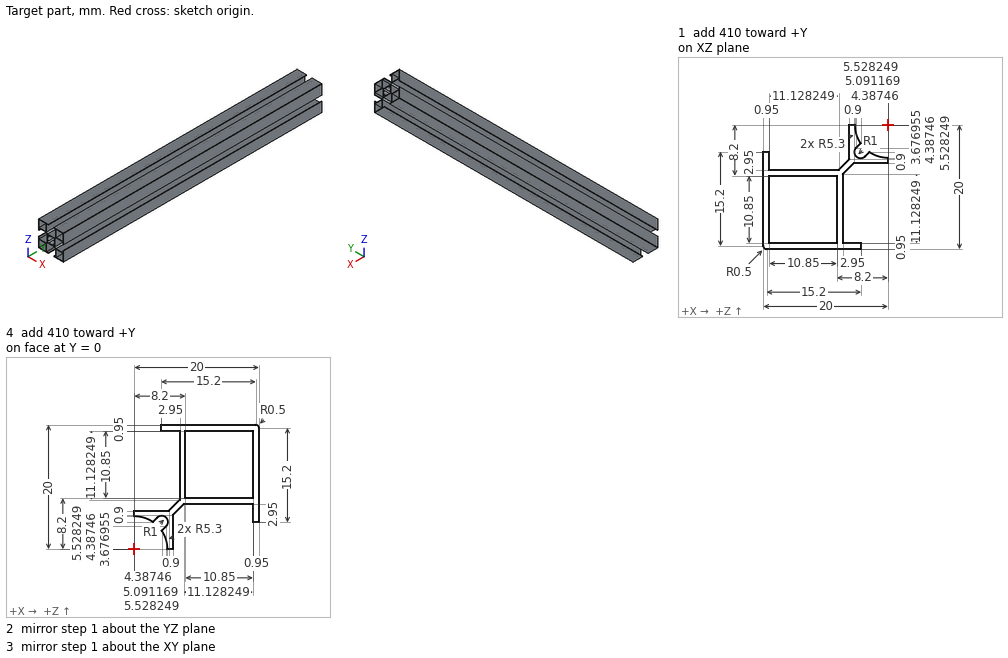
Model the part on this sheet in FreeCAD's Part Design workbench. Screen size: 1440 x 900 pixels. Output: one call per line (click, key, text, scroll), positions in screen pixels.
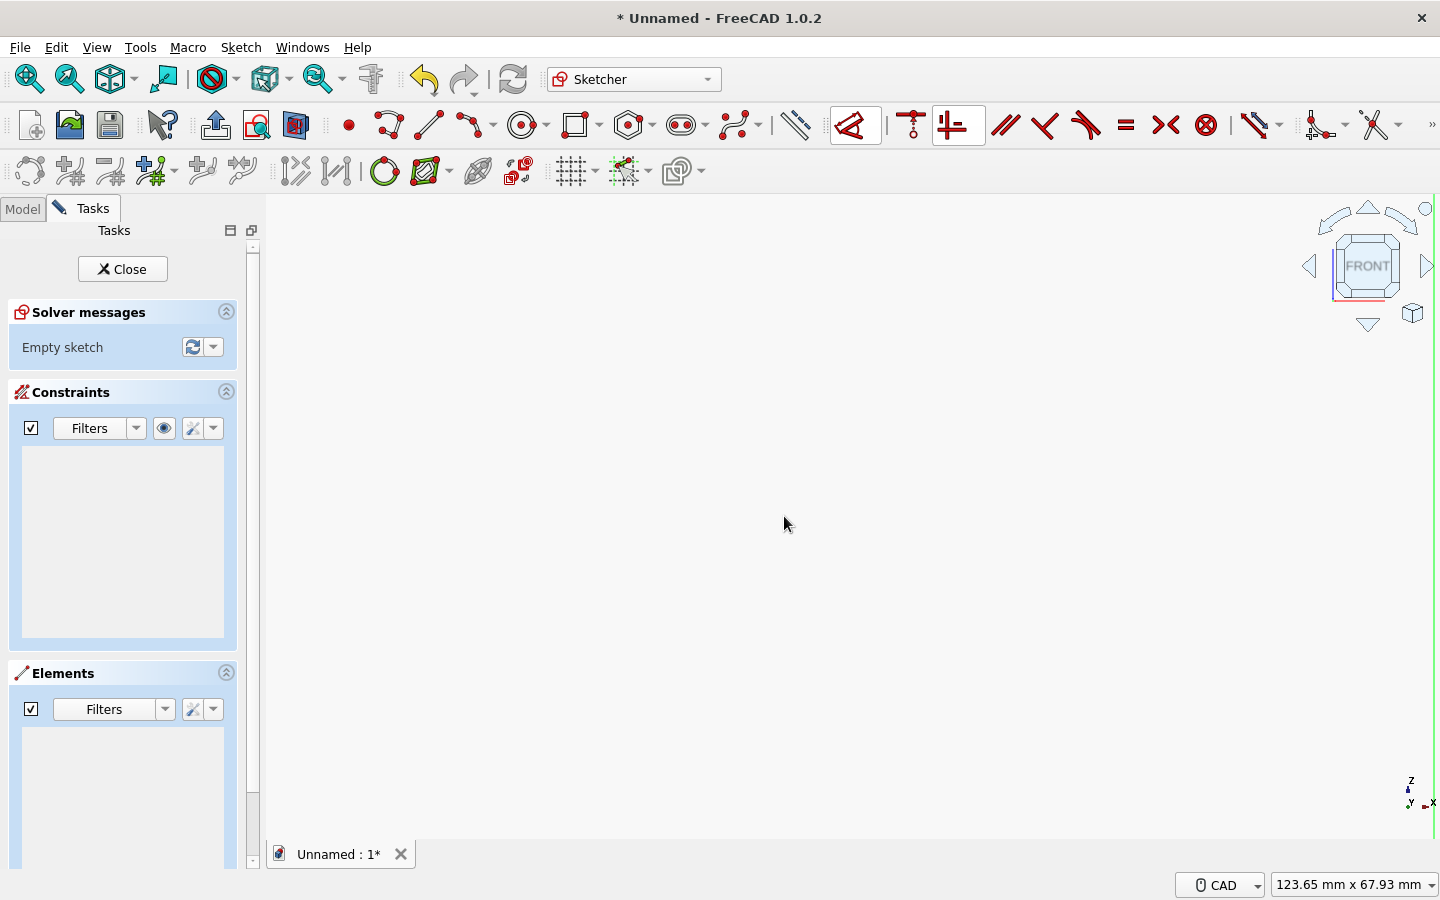
scroll(784, 516, down, 5)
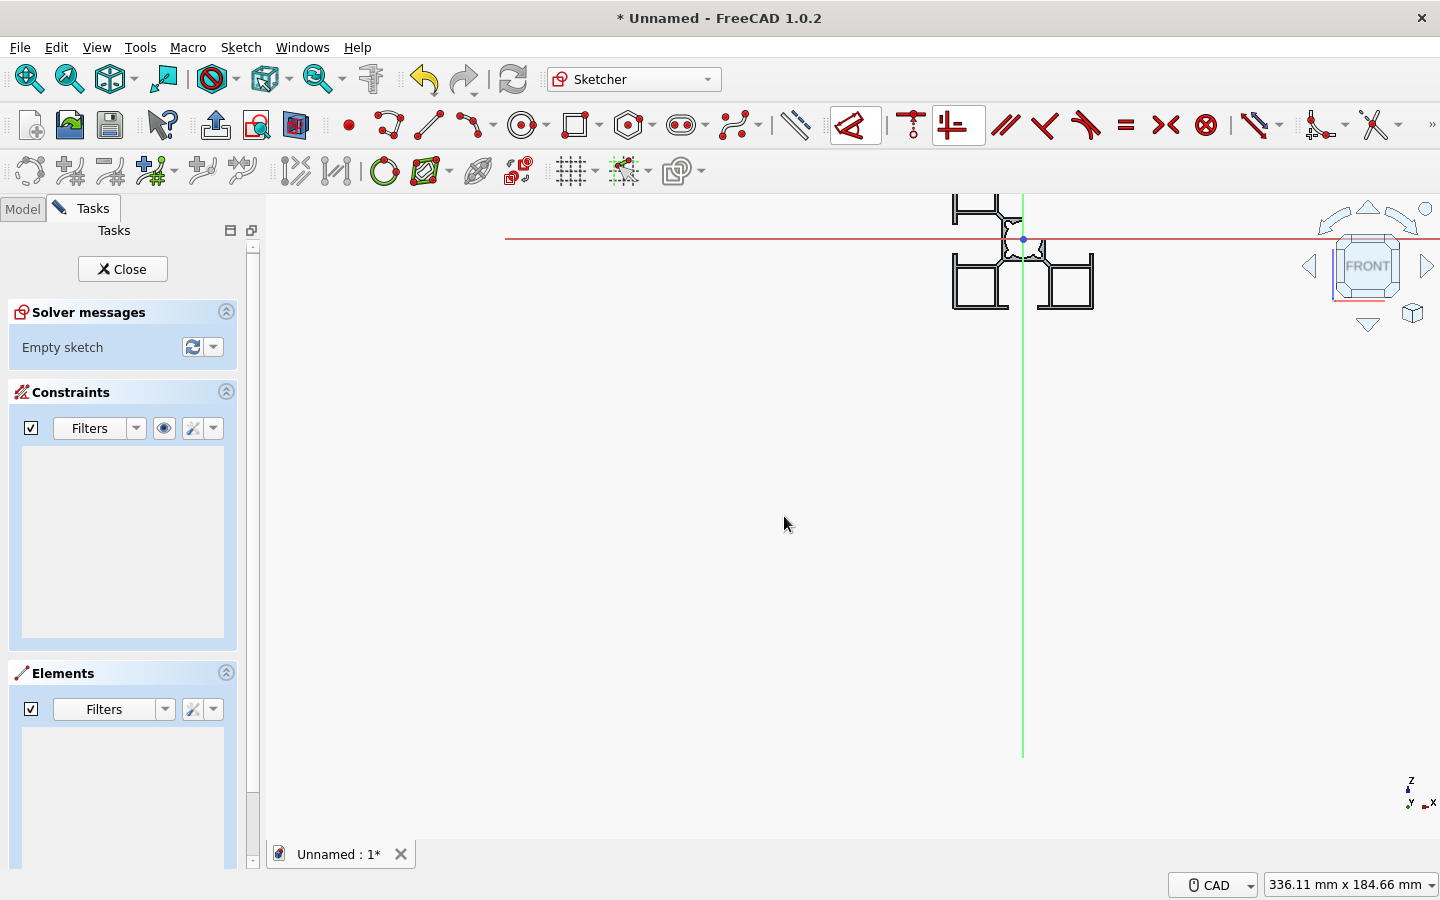
scroll(784, 516, down, 5)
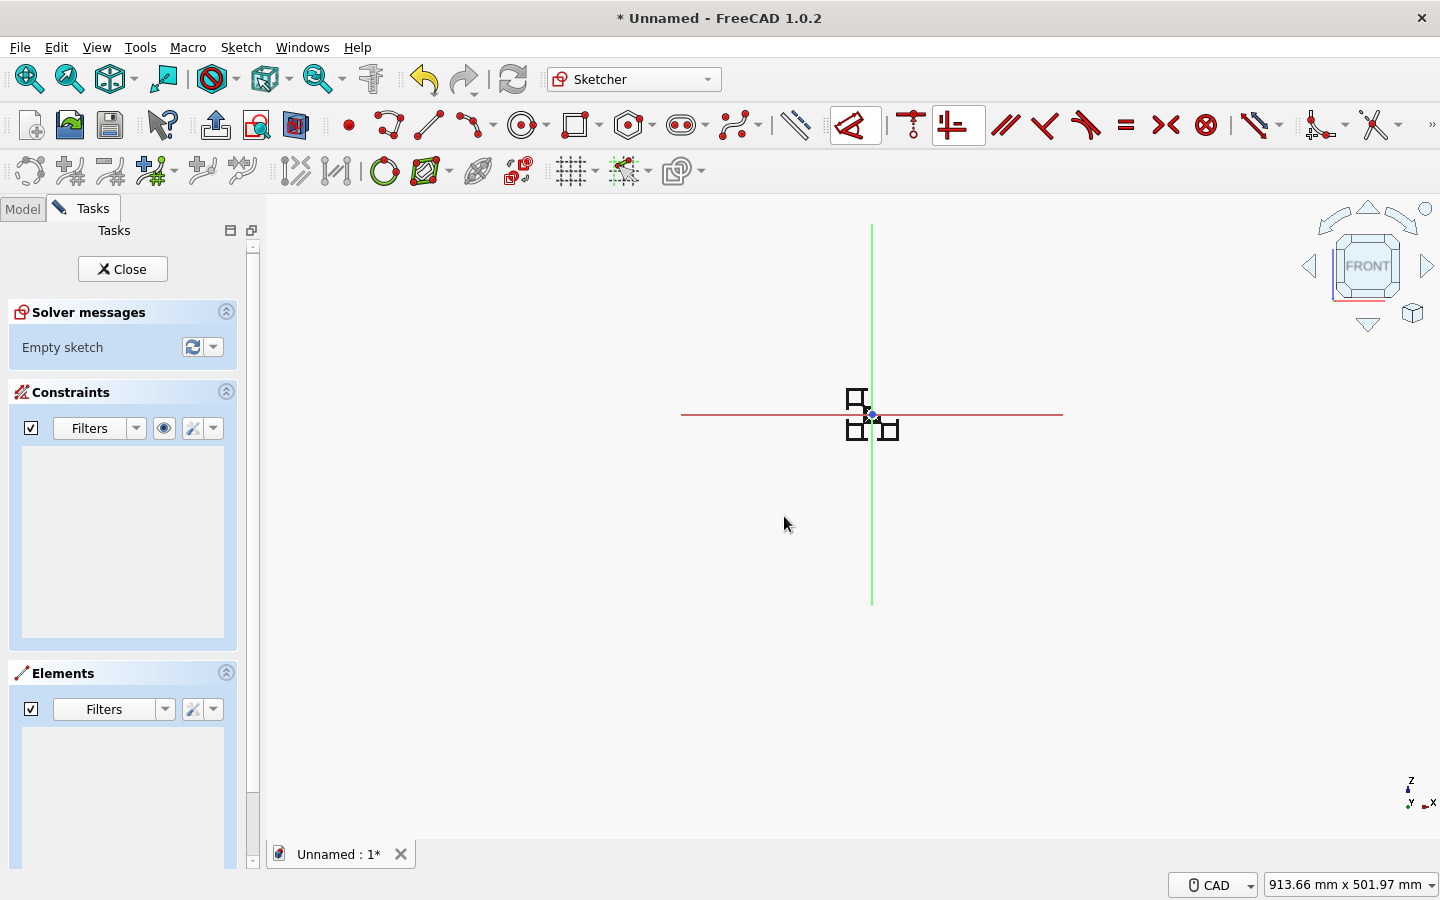
scroll(892, 394, up, 14)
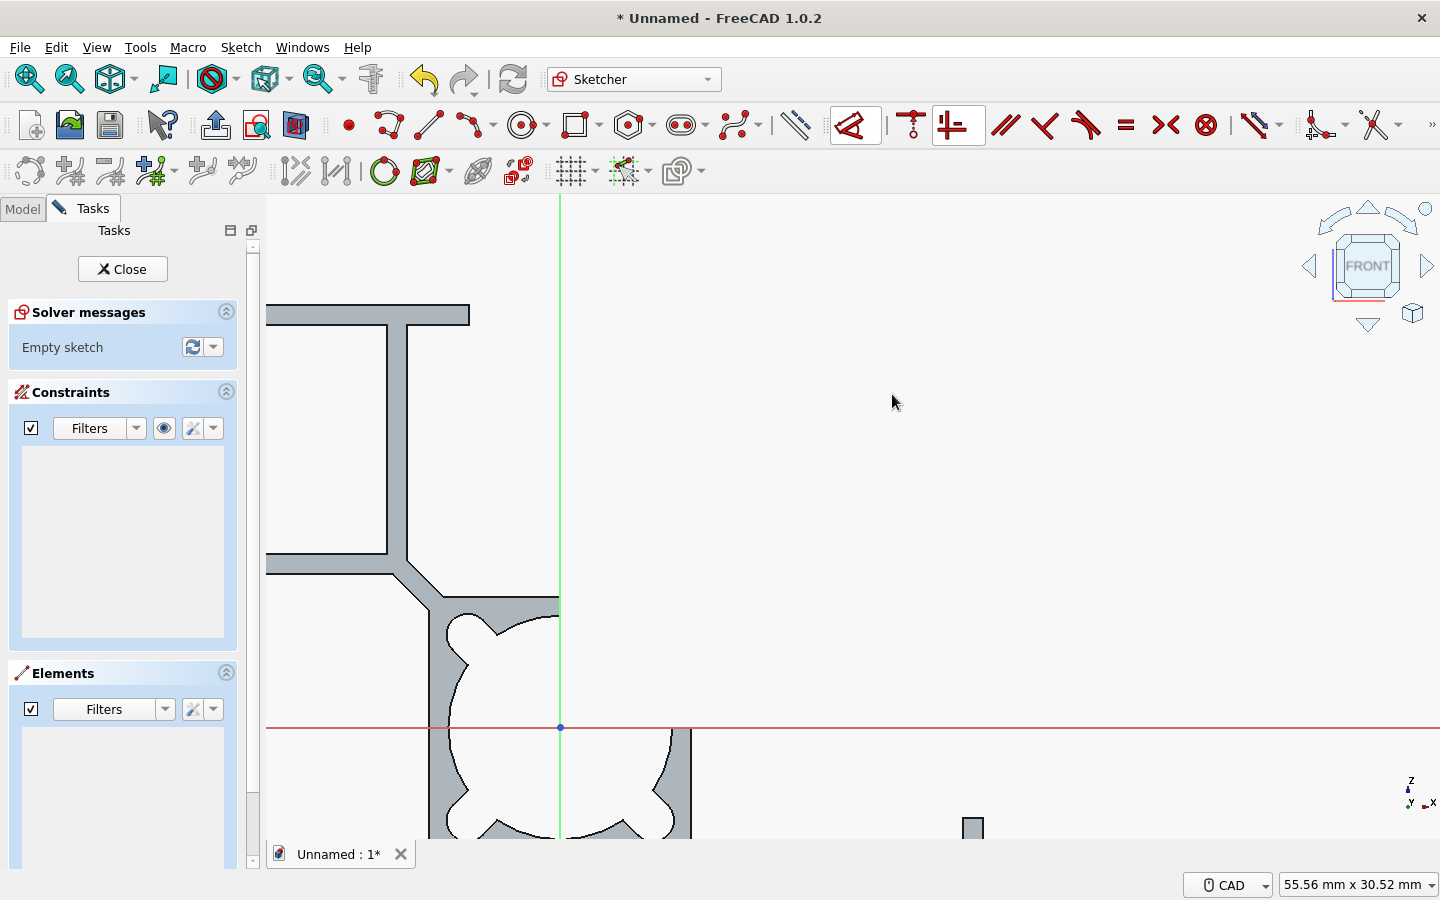
click(390, 126)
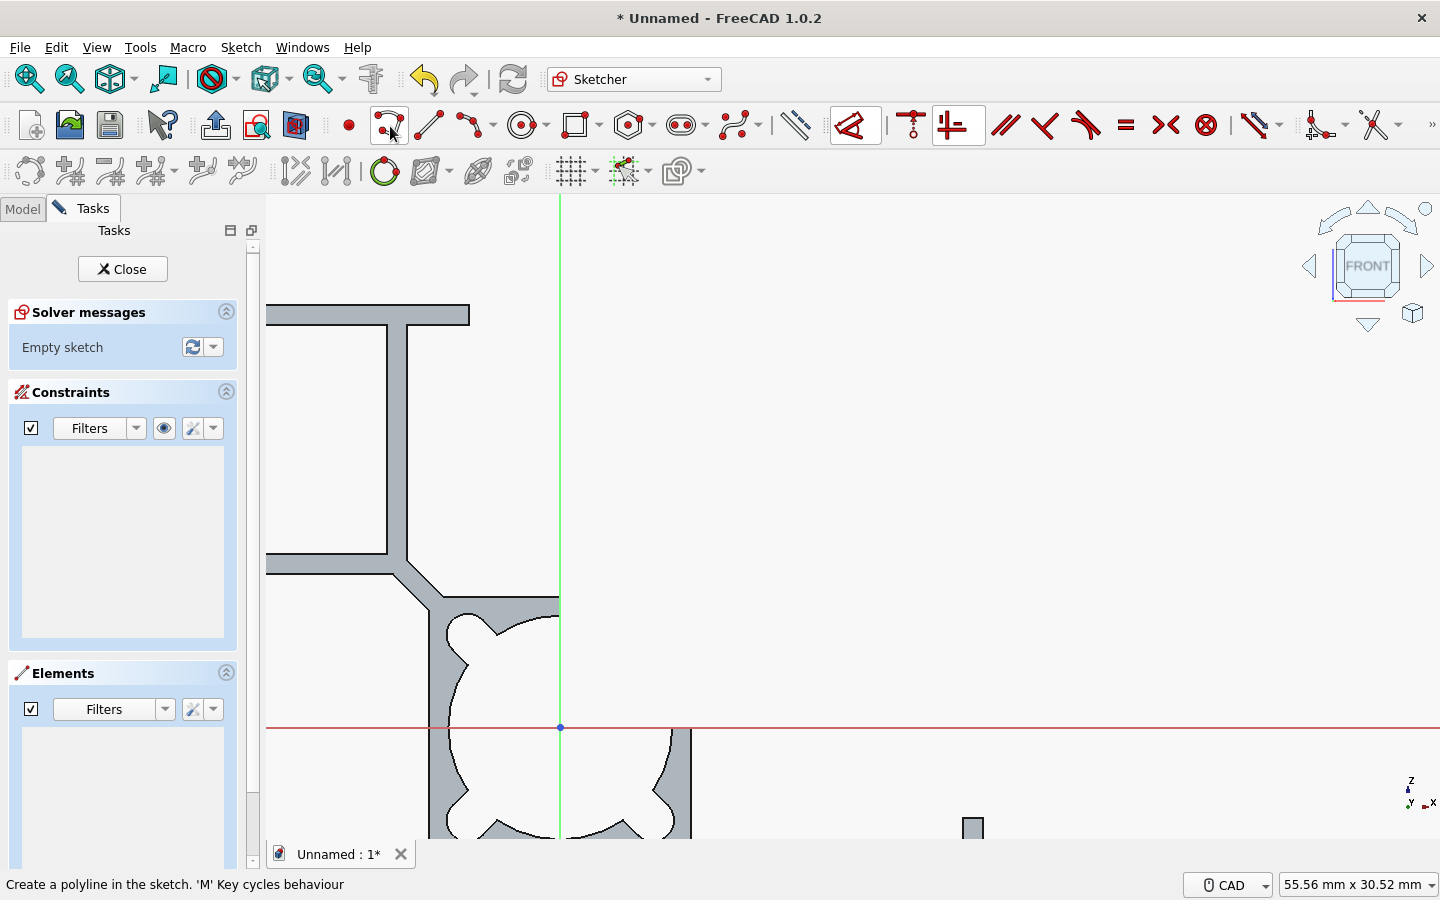
click(983, 316)
click(983, 637)
click(963, 637)
click(963, 574)
click(728, 574)
click(691, 611)
click(691, 728)
click(672, 719)
right_click(672, 719)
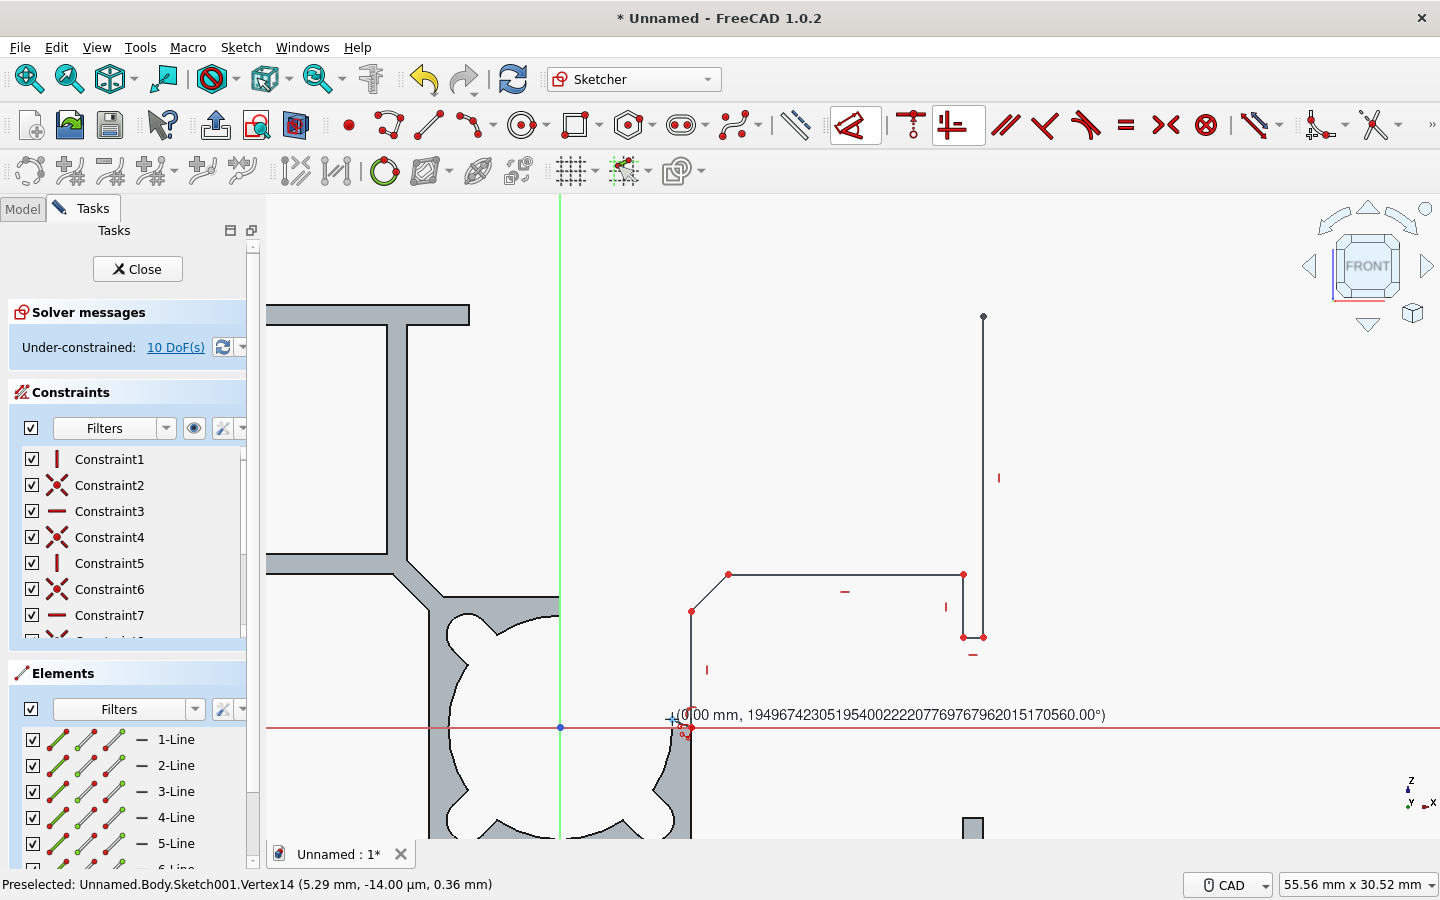
click(430, 126)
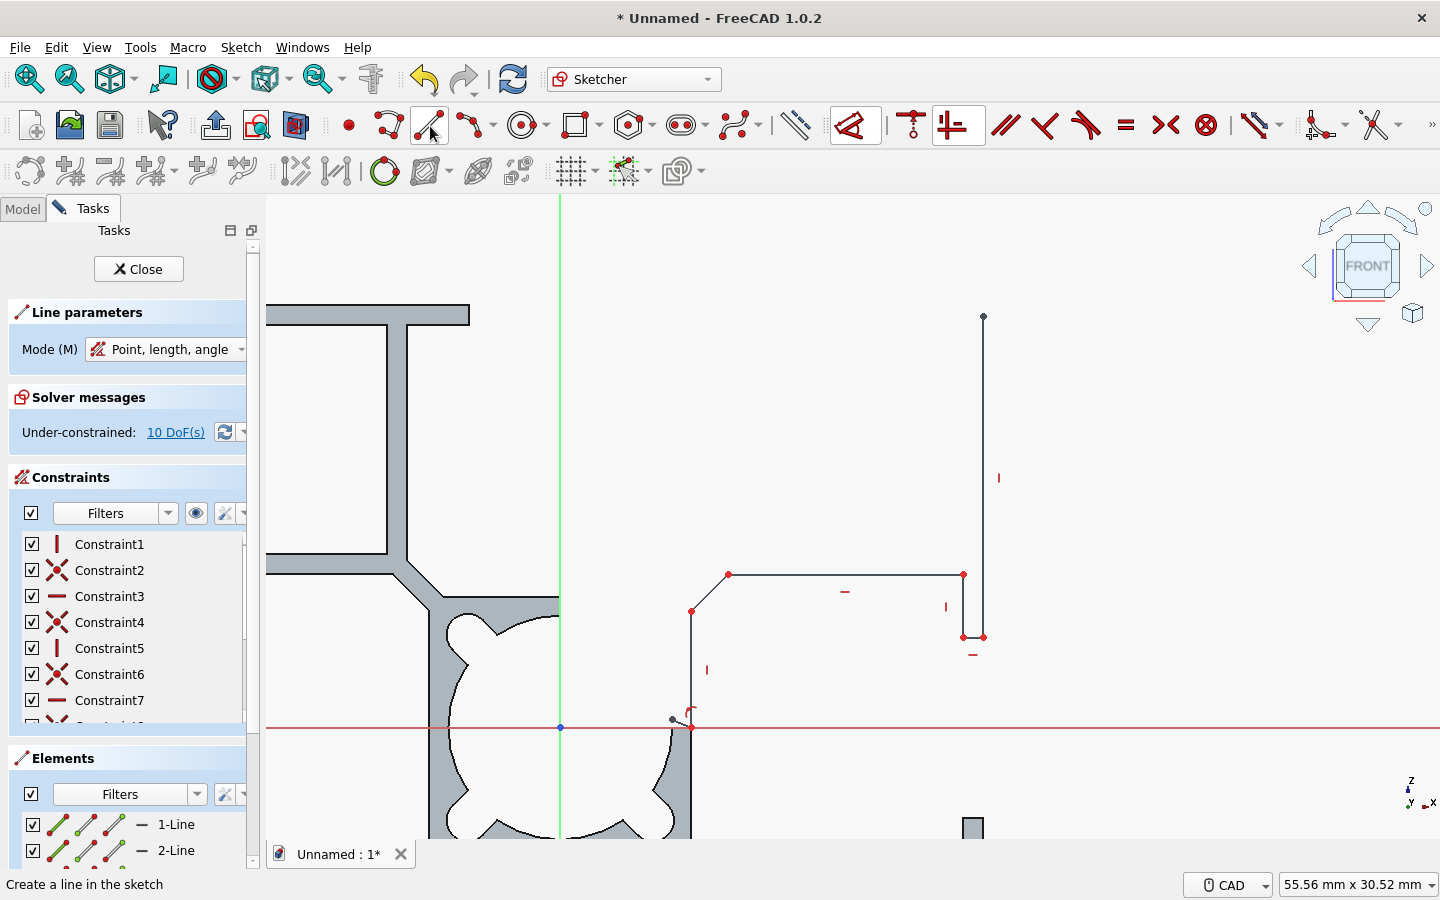
click(653, 665)
click(668, 650)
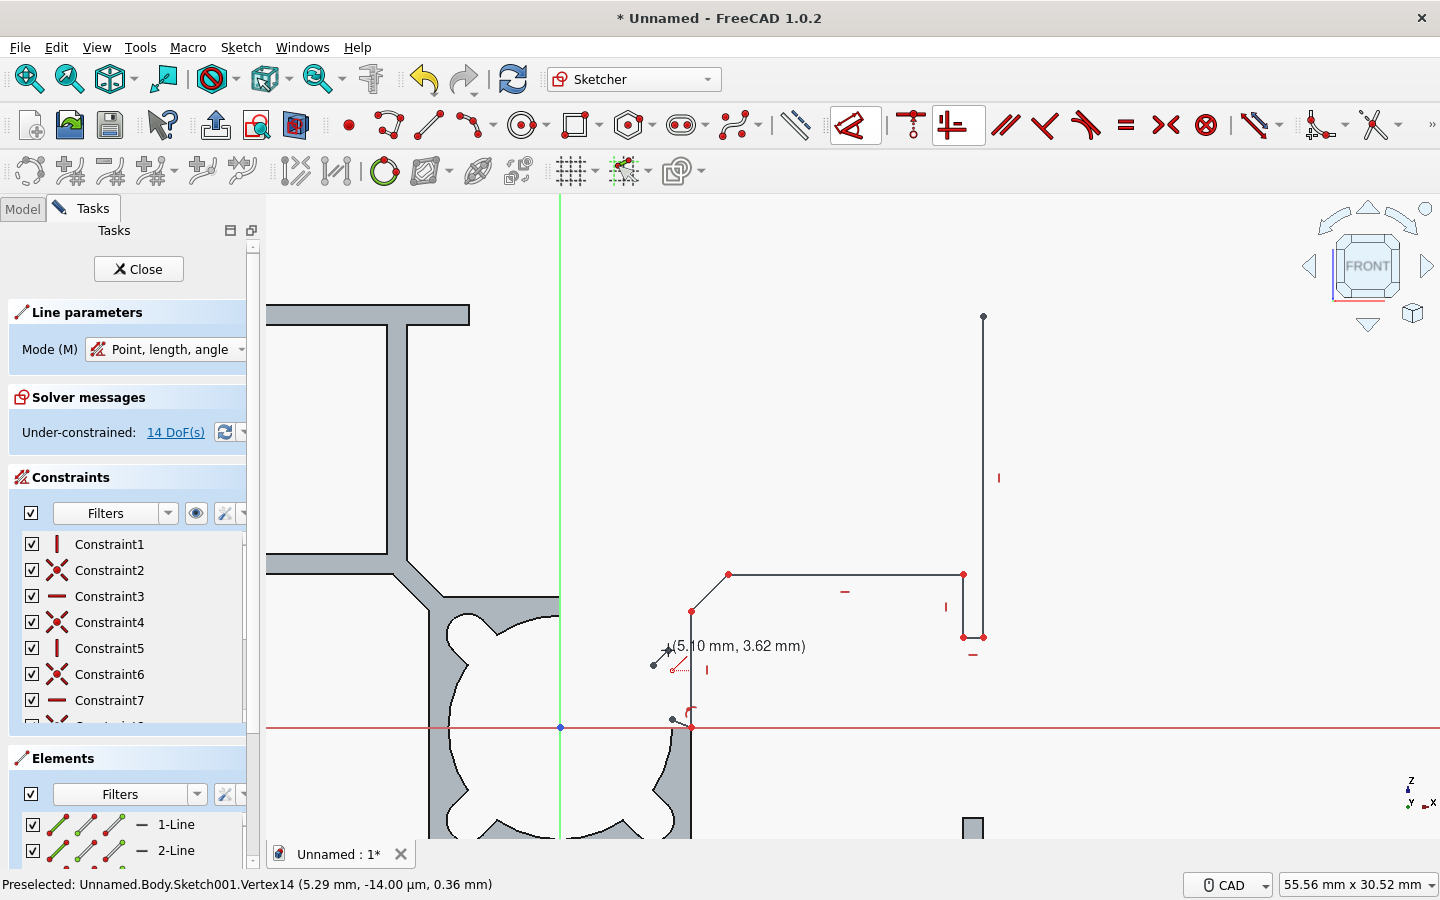
click(638, 620)
click(623, 635)